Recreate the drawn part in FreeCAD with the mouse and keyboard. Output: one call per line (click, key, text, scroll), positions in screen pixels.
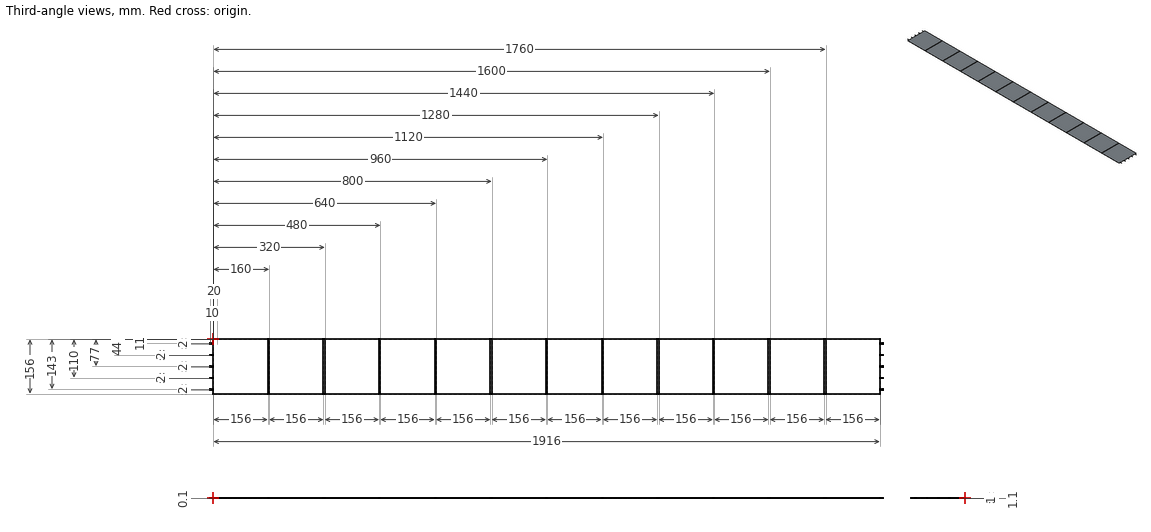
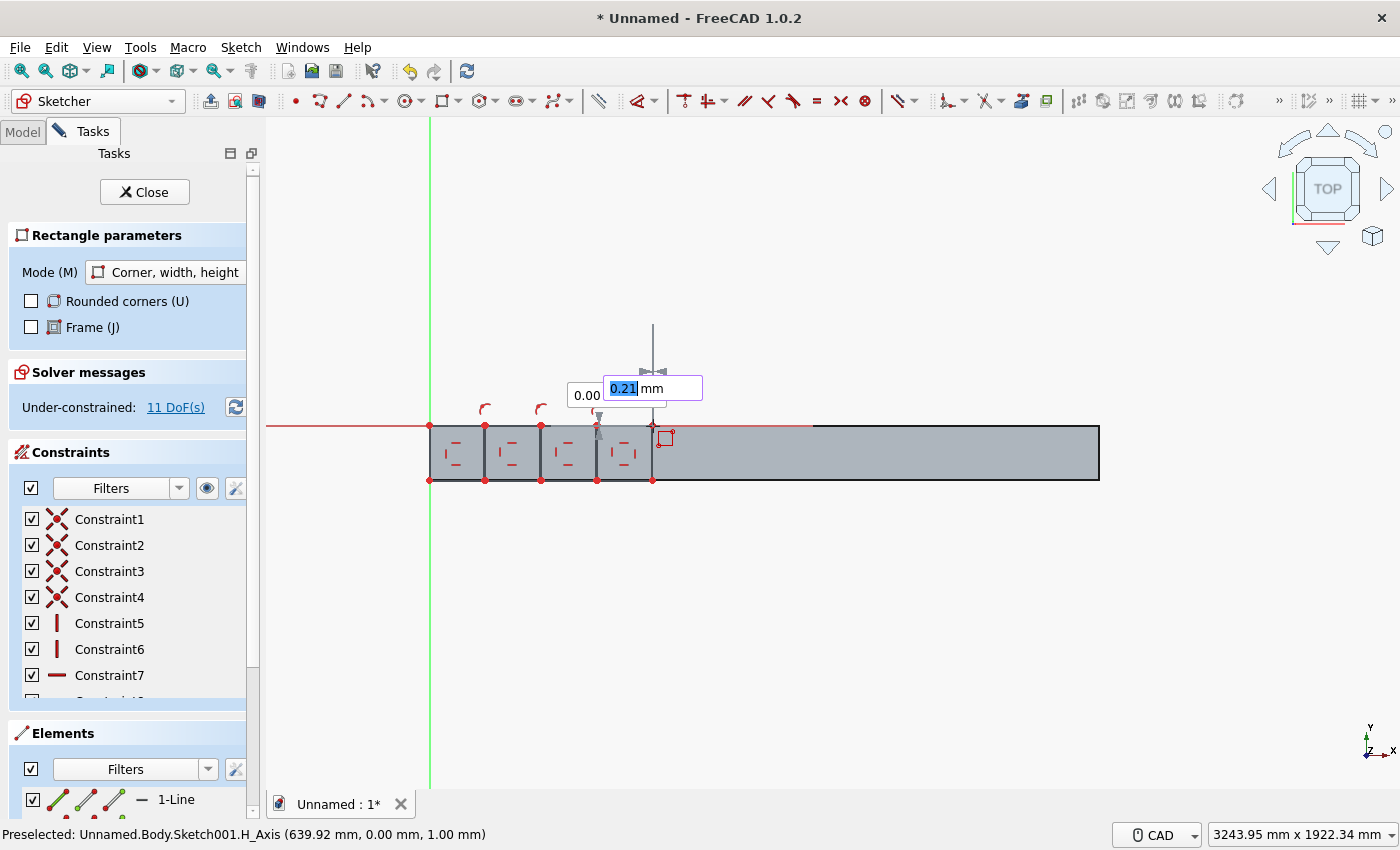
click(708, 480)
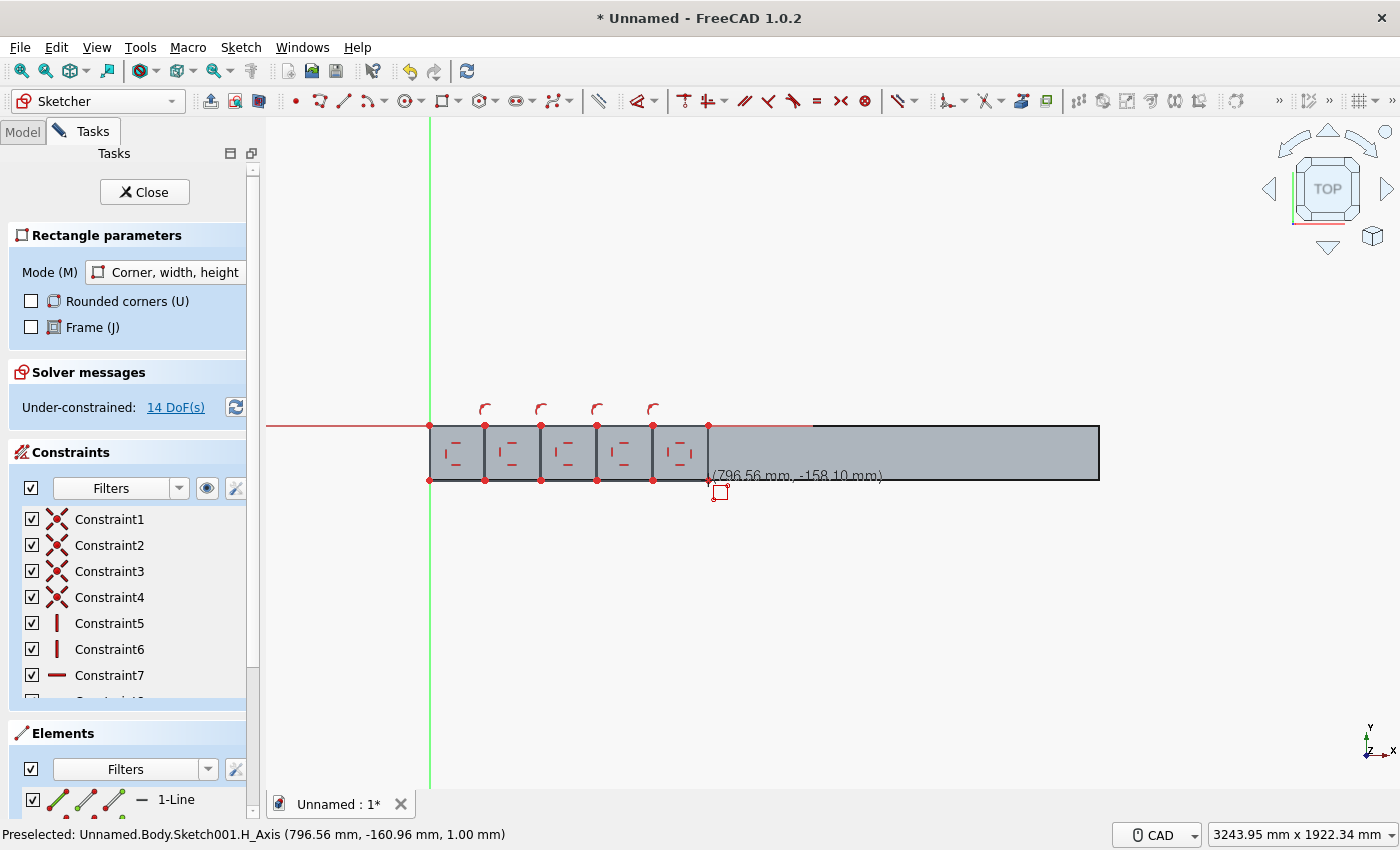
scroll(709, 426, up, 13)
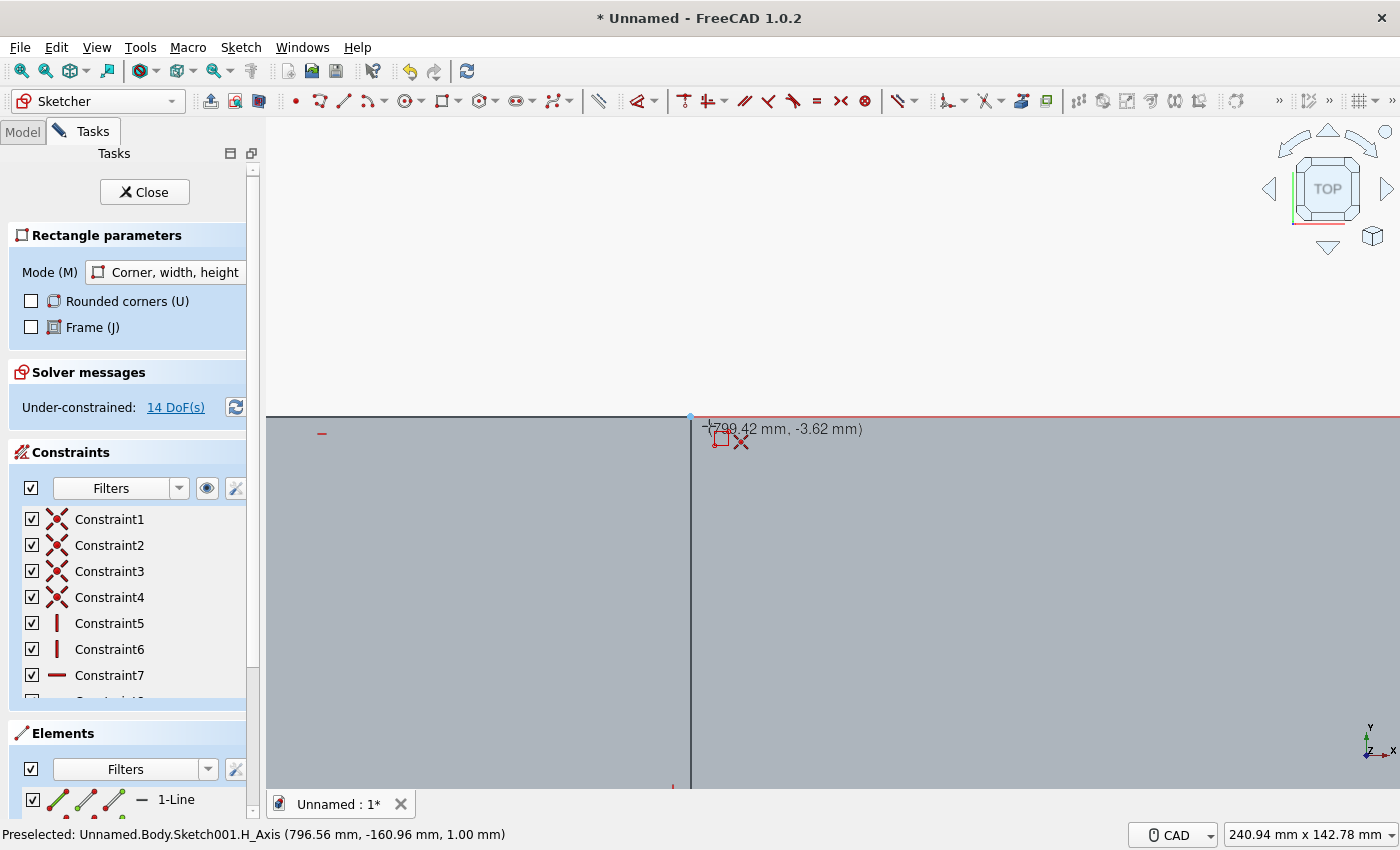
click(707, 417)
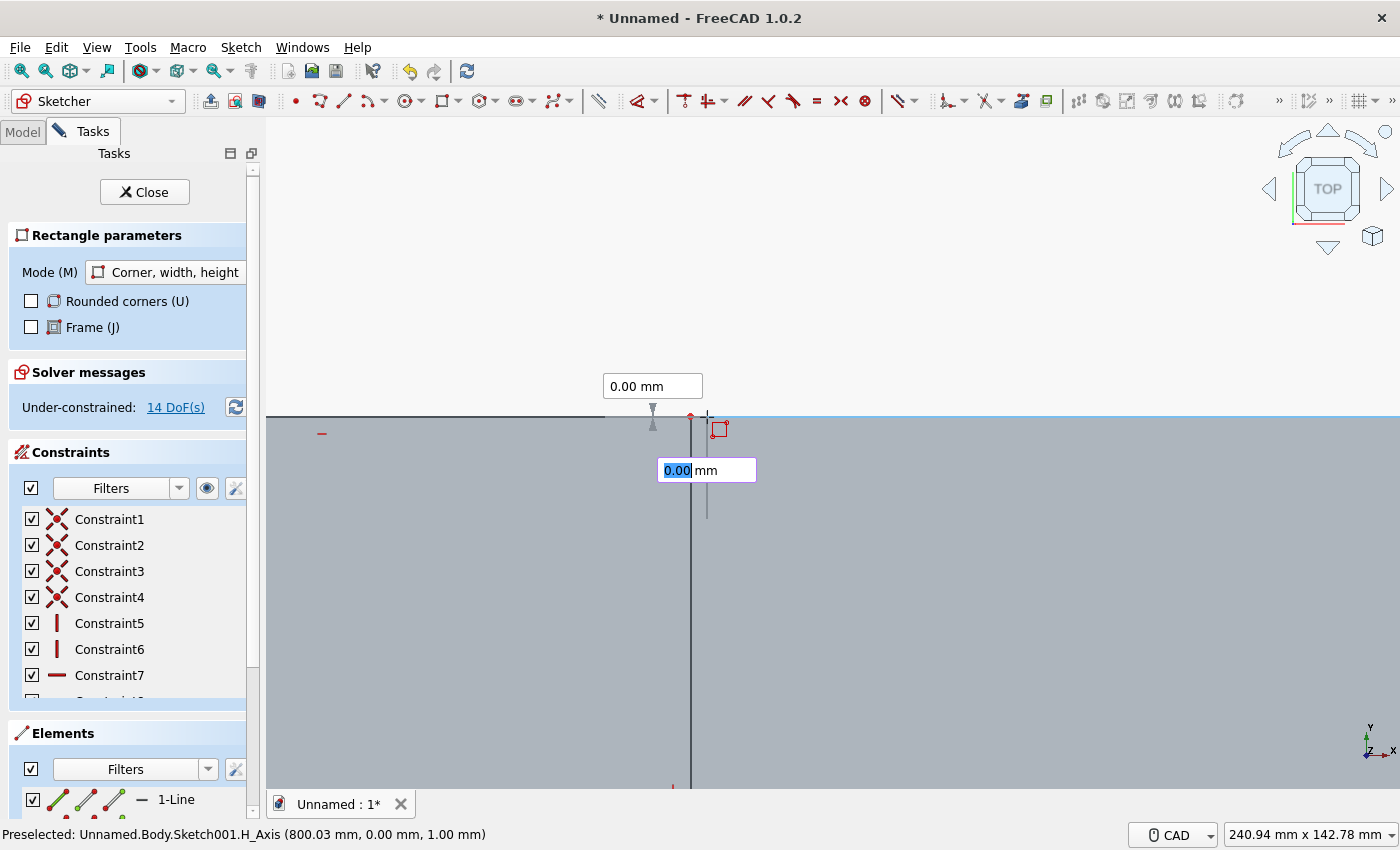
scroll(709, 426, down, 13)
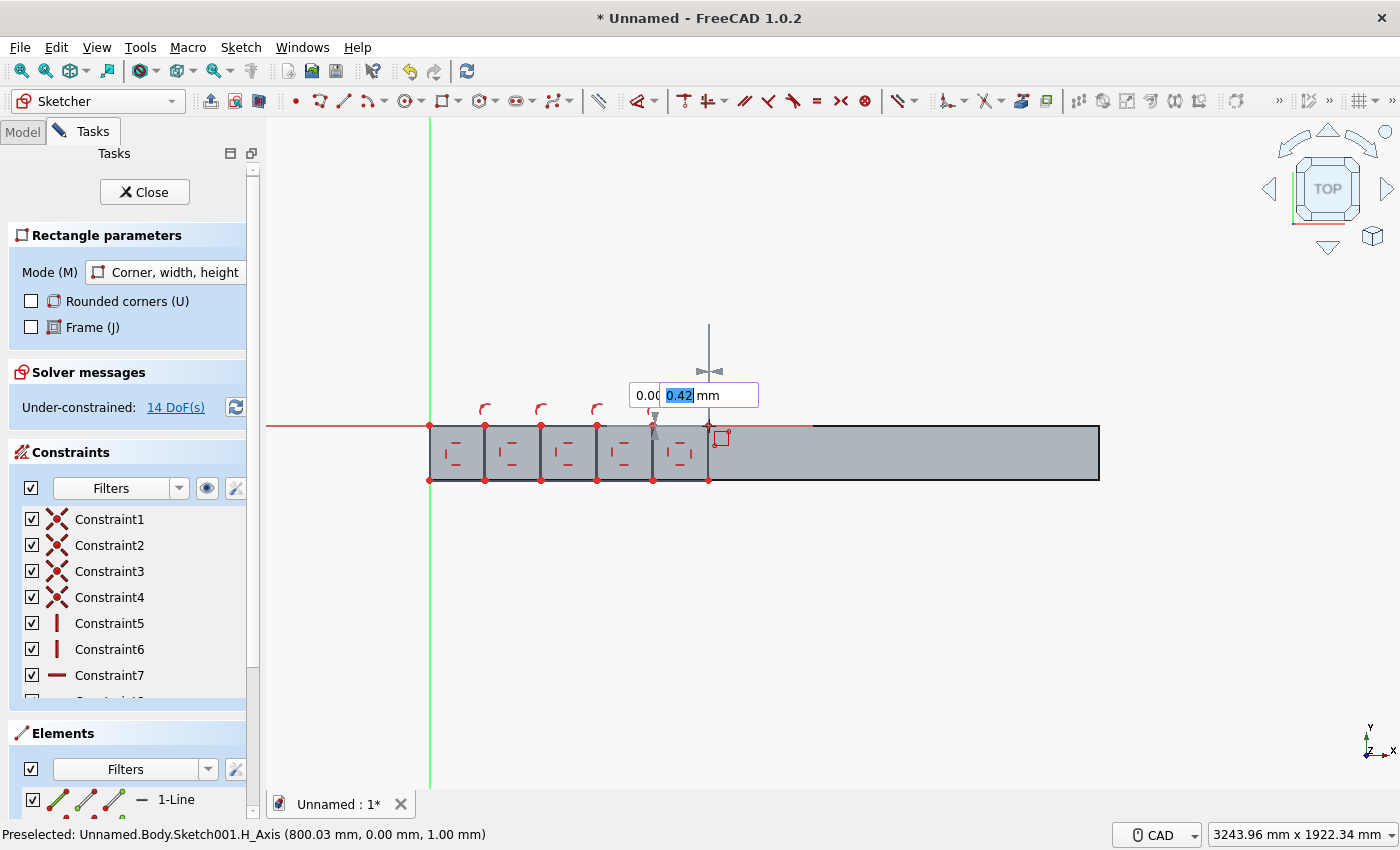
click(764, 480)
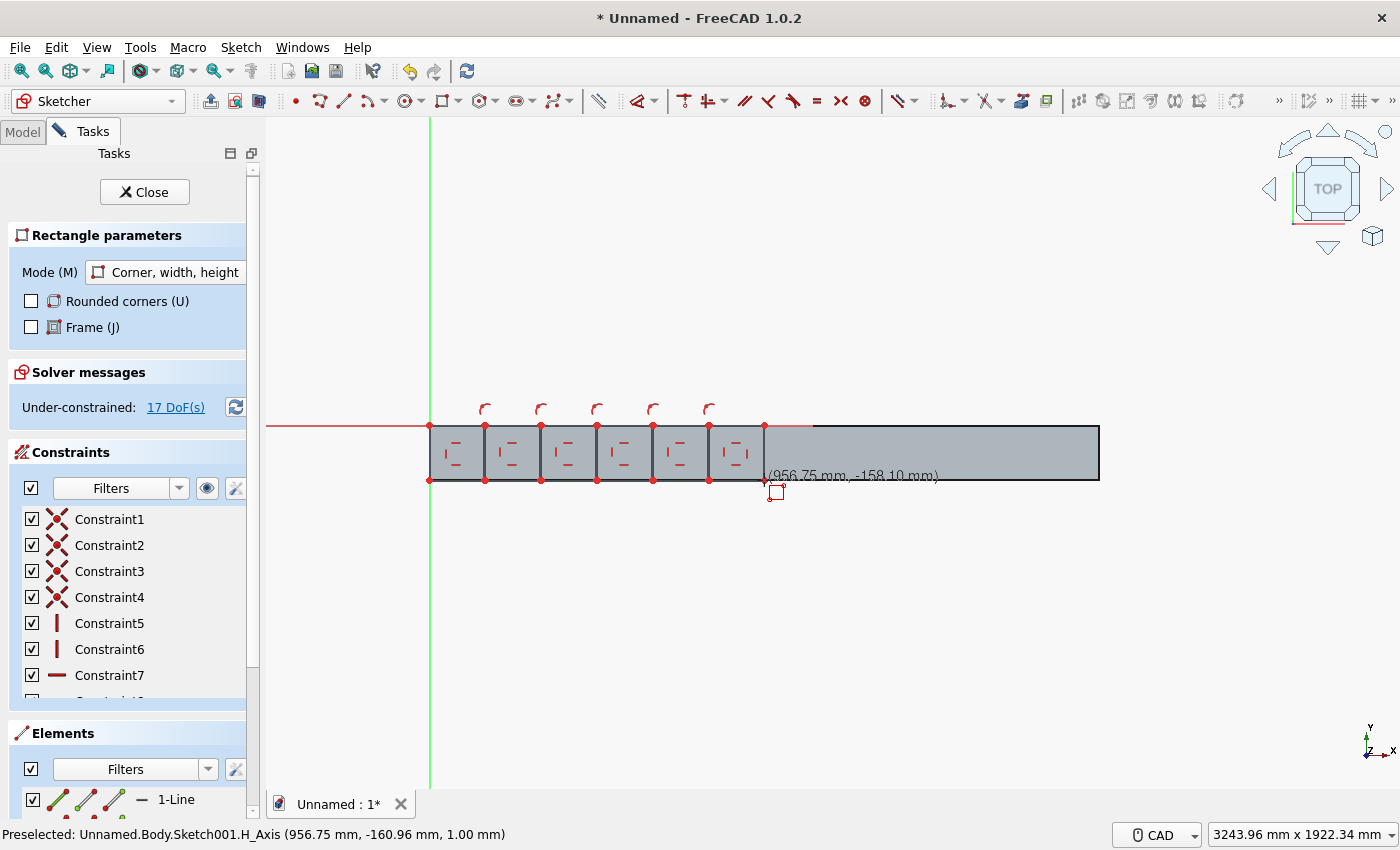
scroll(765, 426, up, 13)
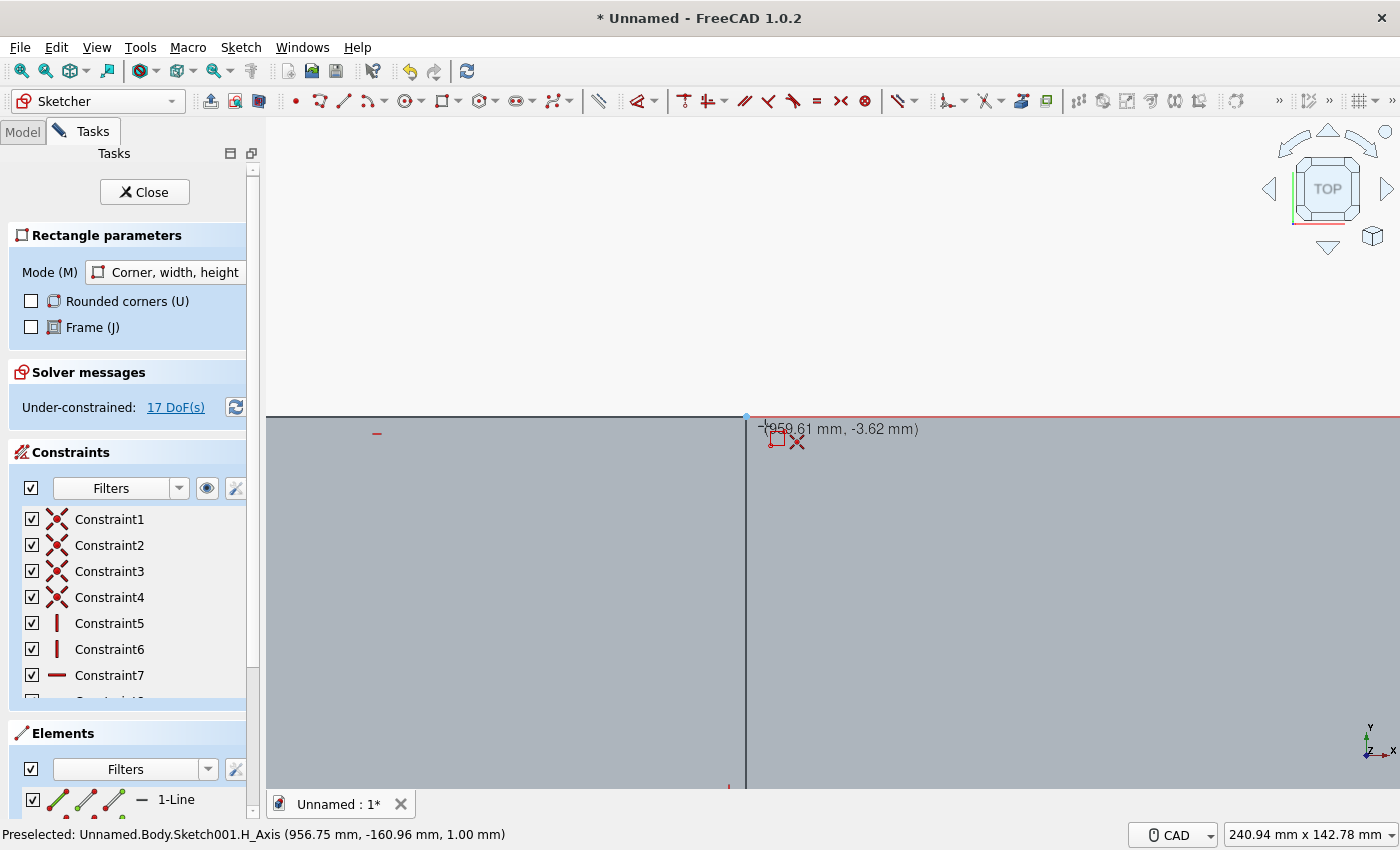
click(761, 417)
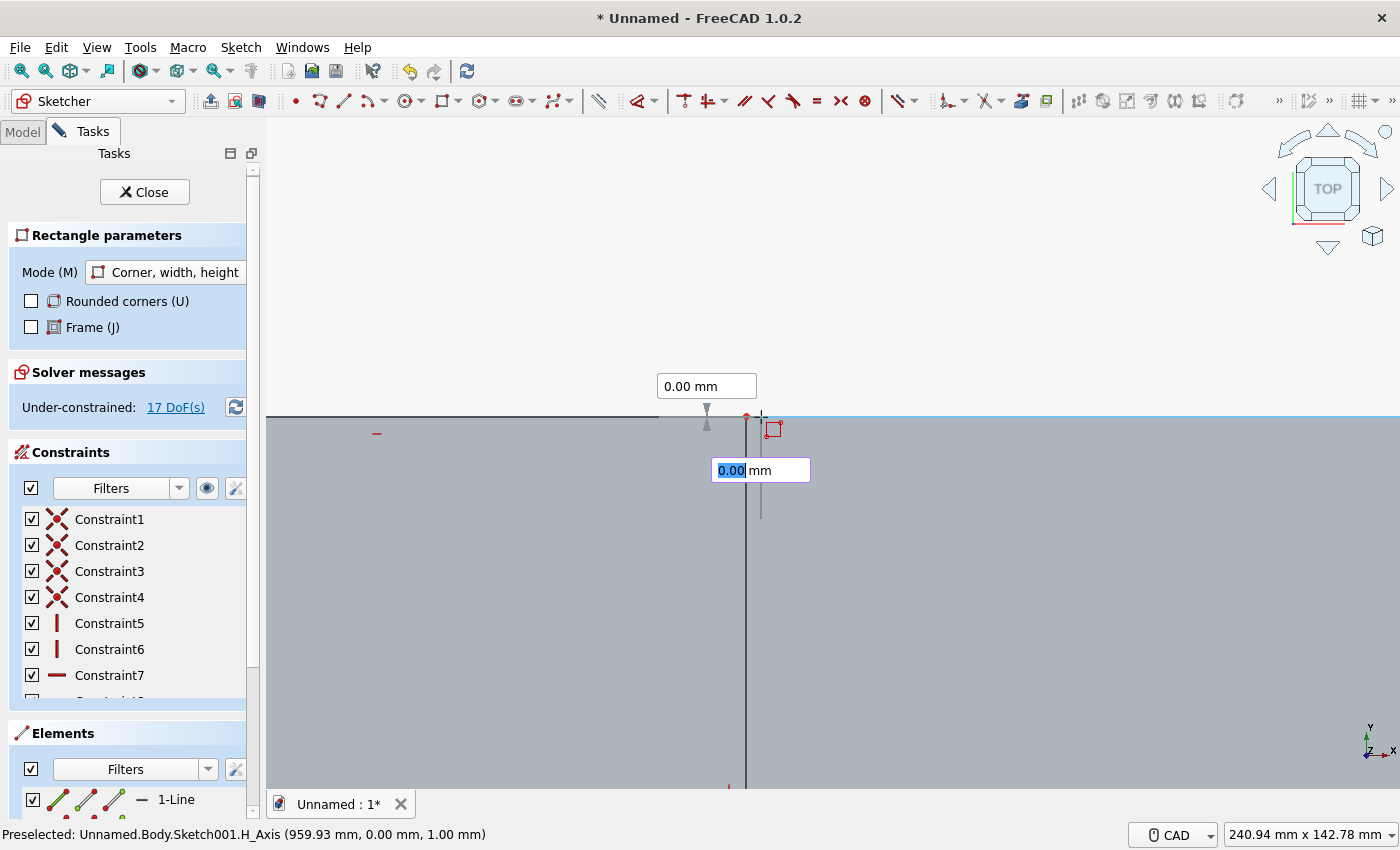
scroll(766, 426, down, 13)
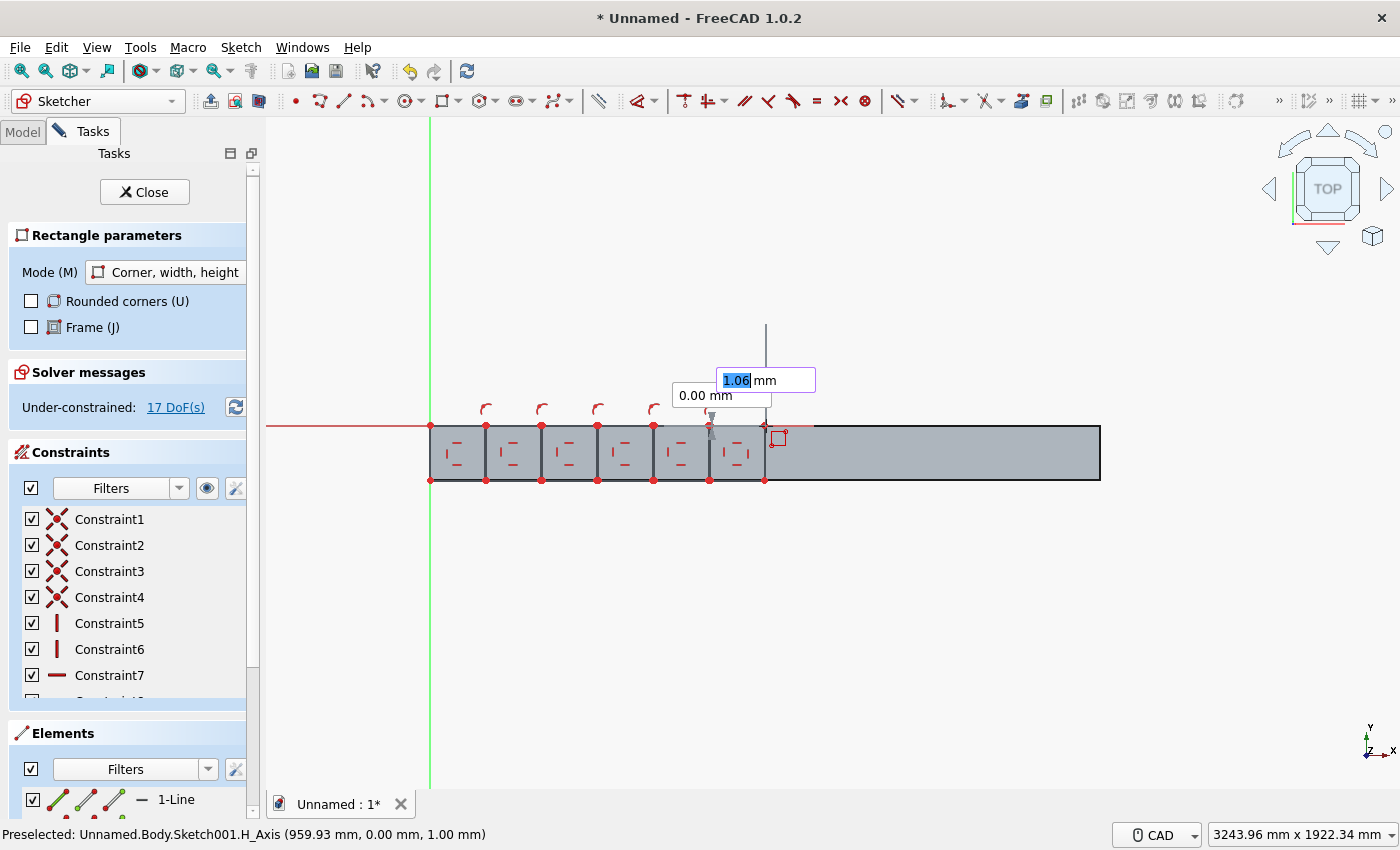
click(821, 480)